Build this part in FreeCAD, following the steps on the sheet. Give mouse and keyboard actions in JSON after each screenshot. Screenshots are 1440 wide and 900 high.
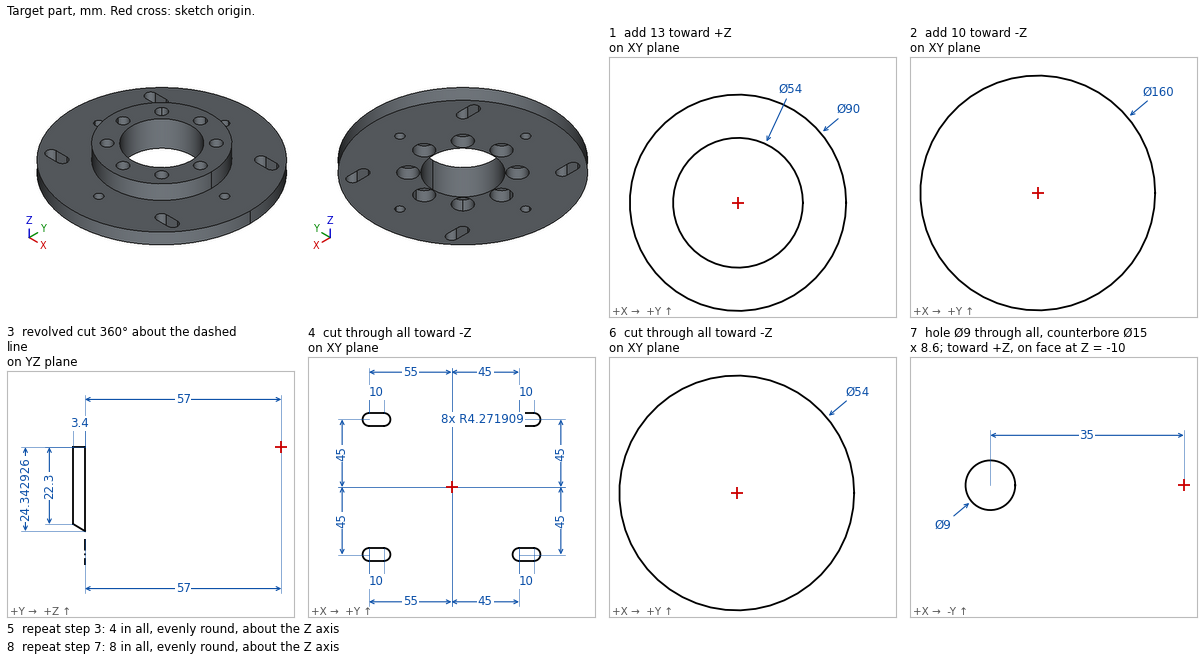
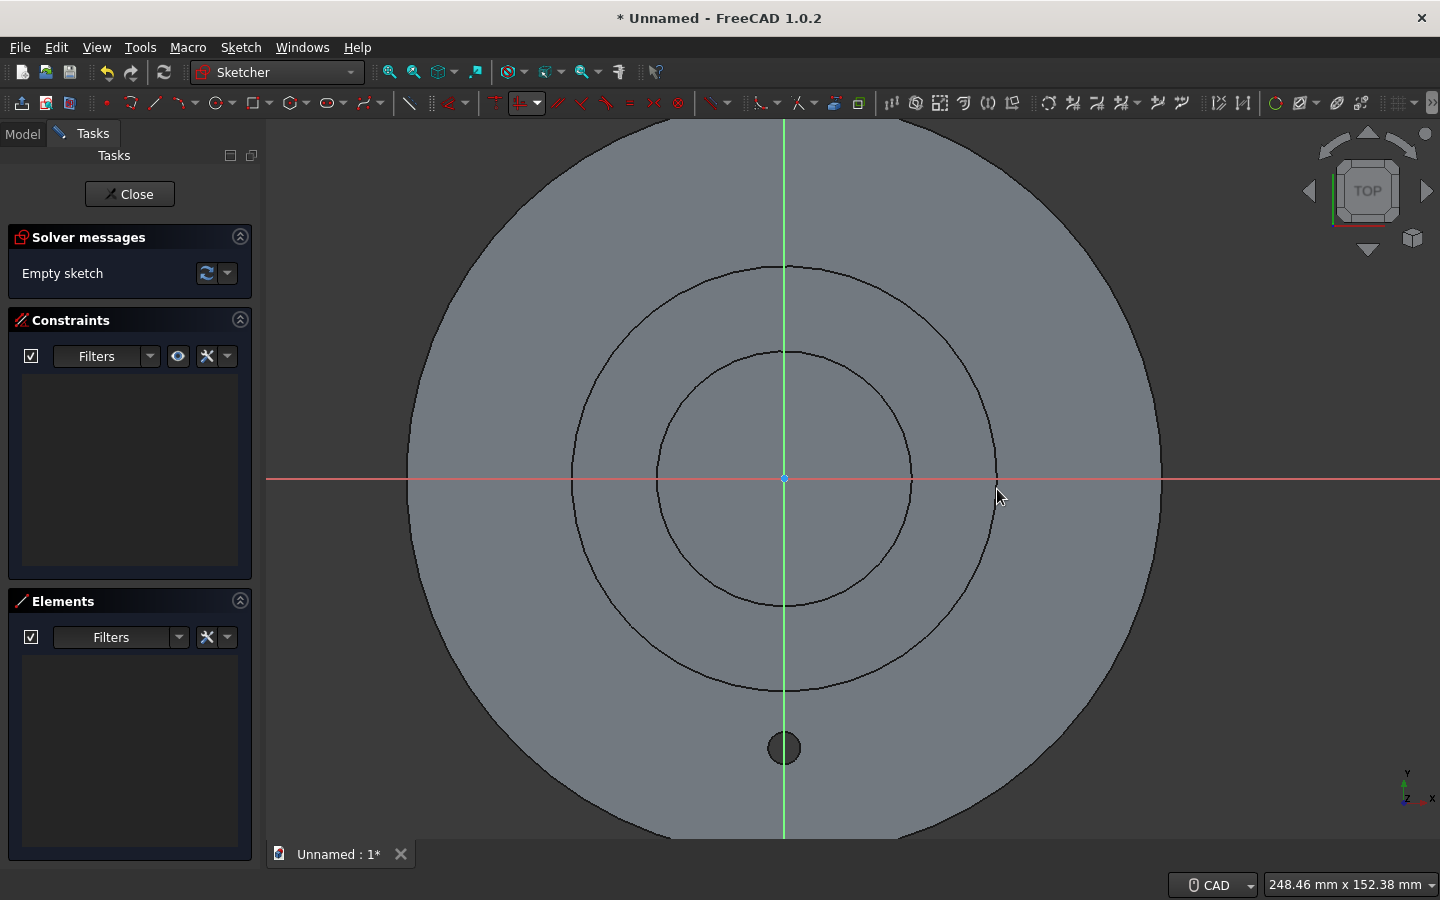
{"action": "left_click", "coordinate": [997, 266]}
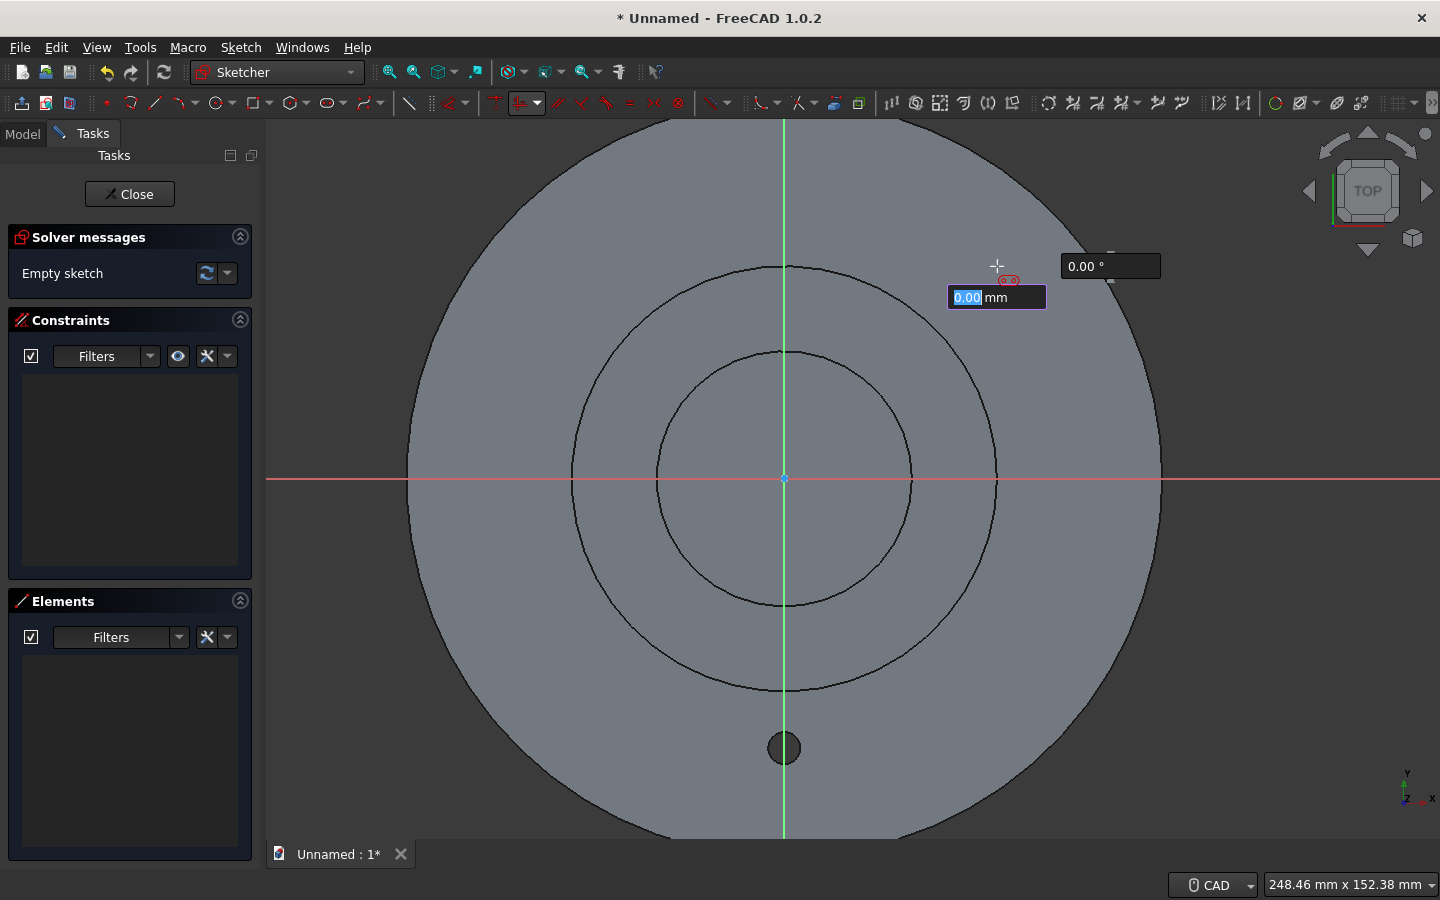
{"action": "left_click", "coordinate": [1044, 266]}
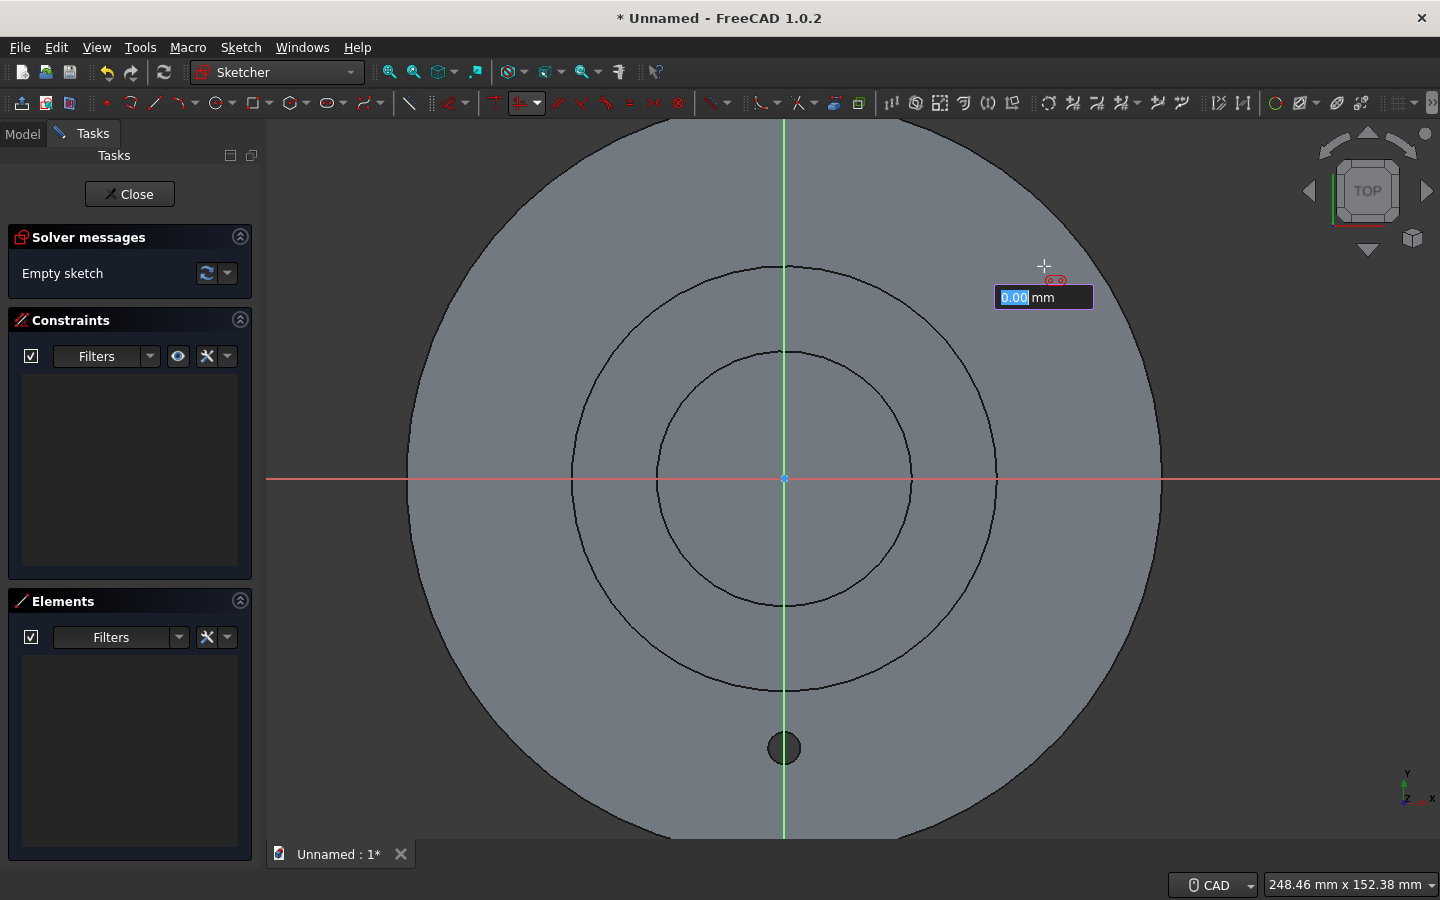
{"action": "left_click", "coordinate": [1021, 246]}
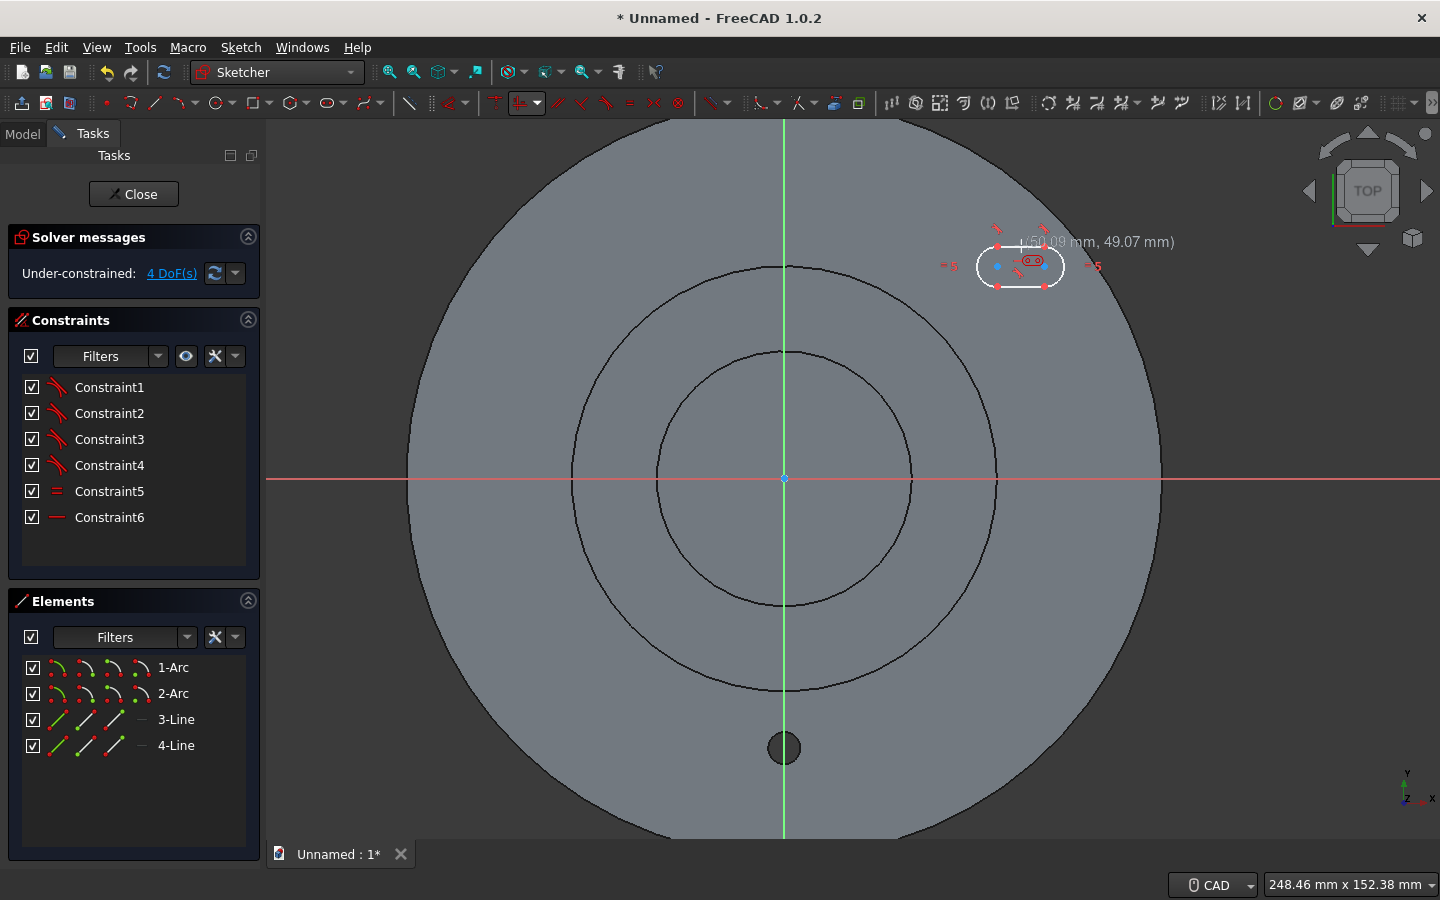
{"action": "left_click", "coordinate": [997, 691]}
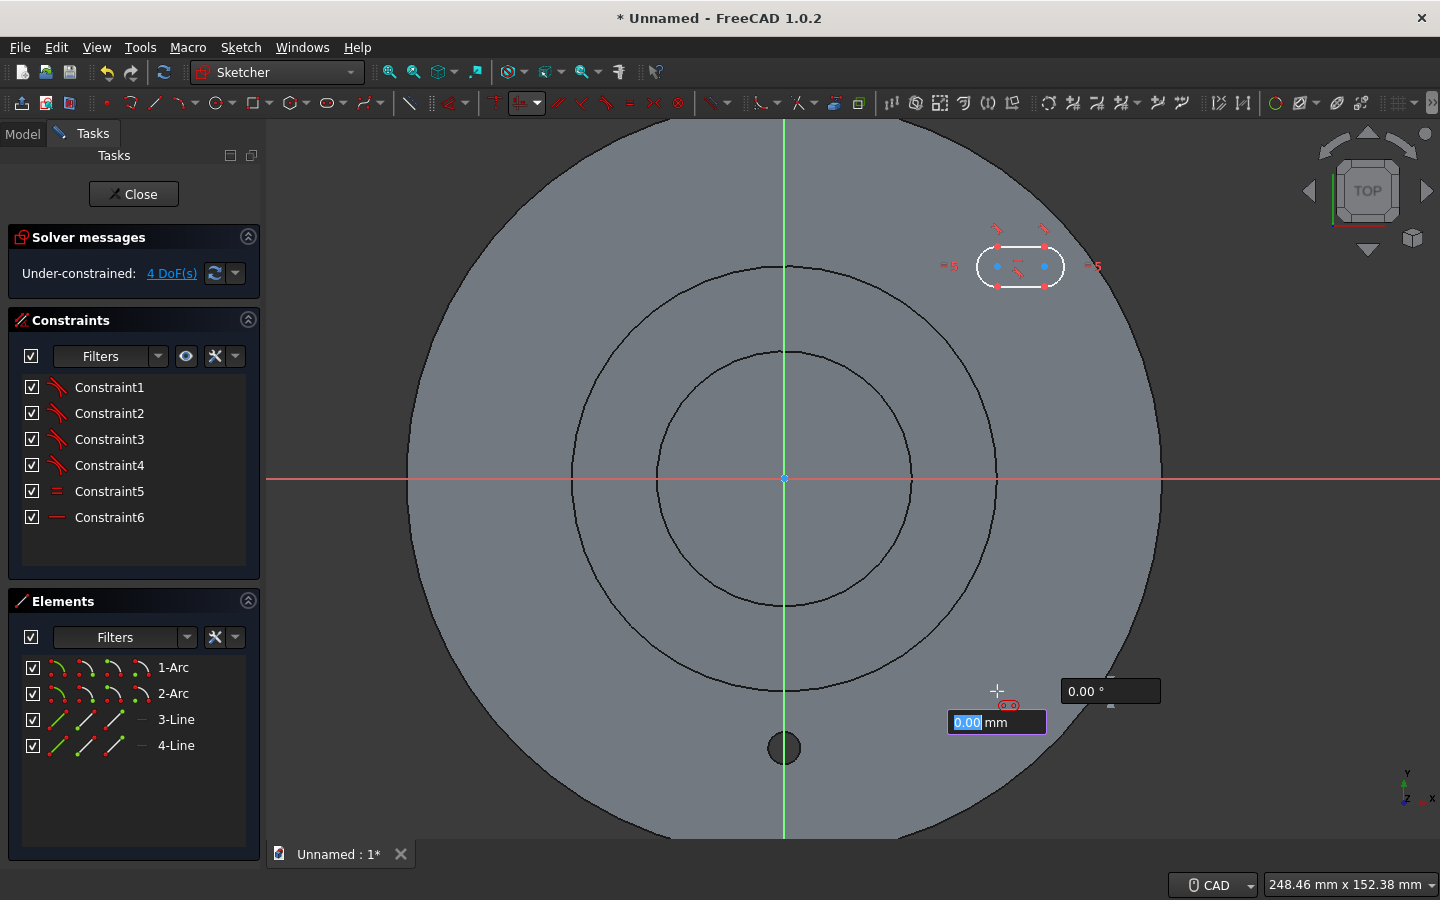
{"action": "left_click", "coordinate": [1044, 691]}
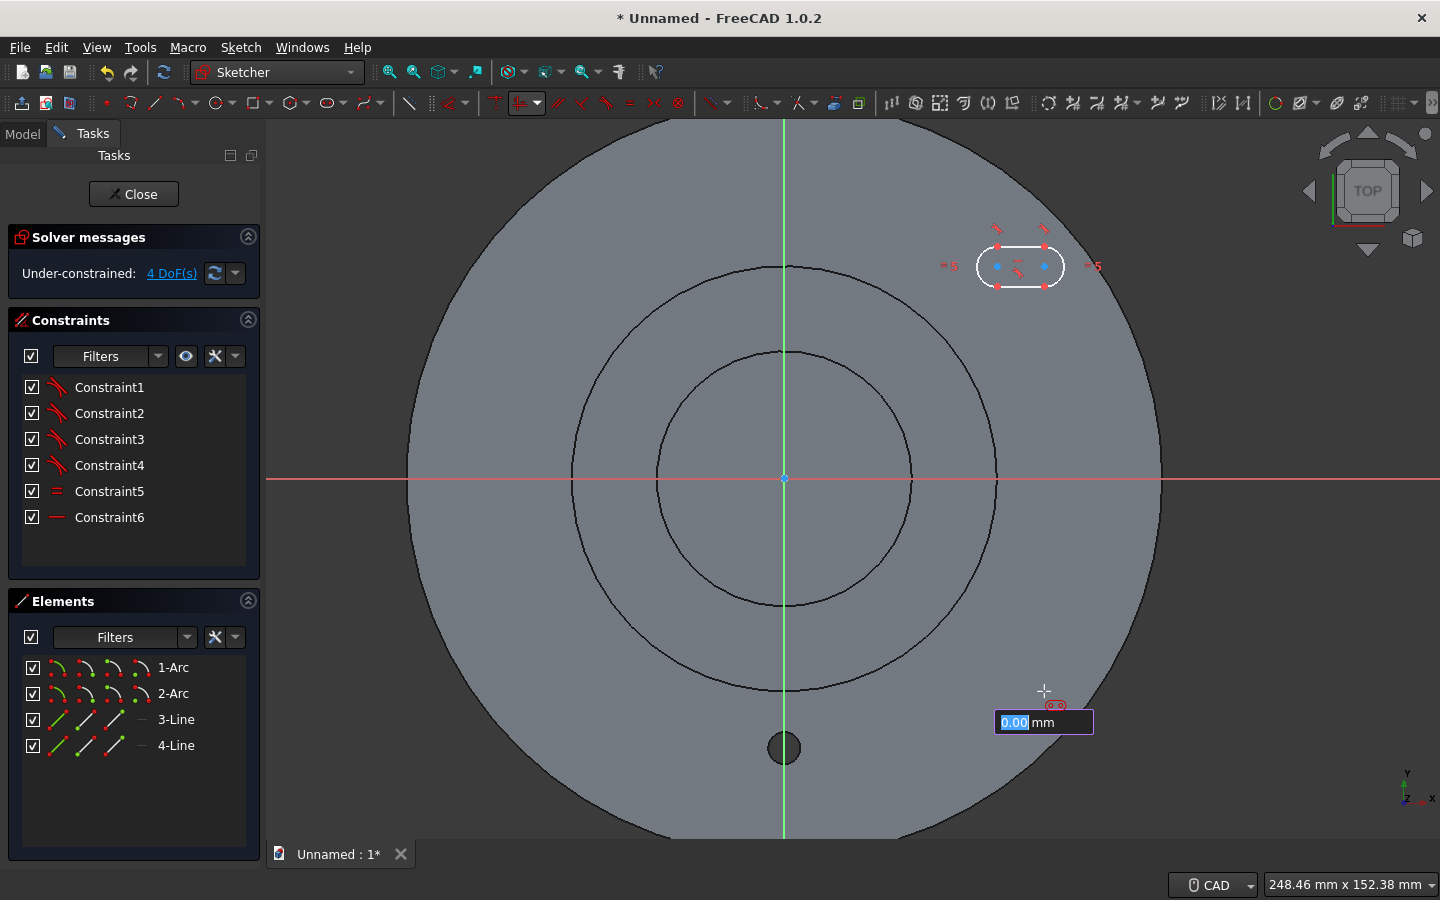
{"action": "left_click", "coordinate": [1021, 671]}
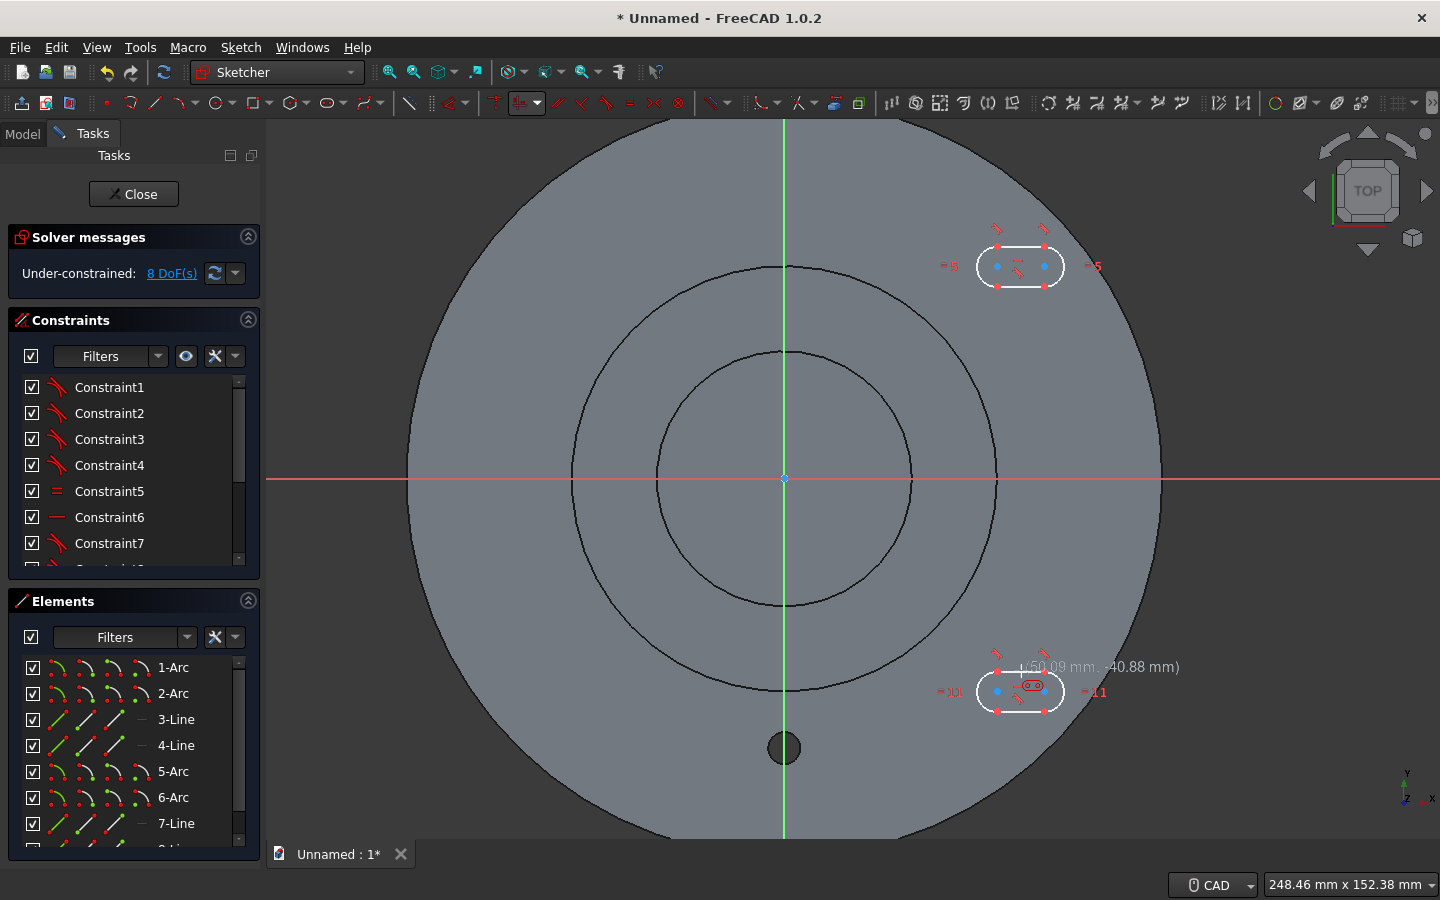
{"action": "left_click", "coordinate": [524, 691]}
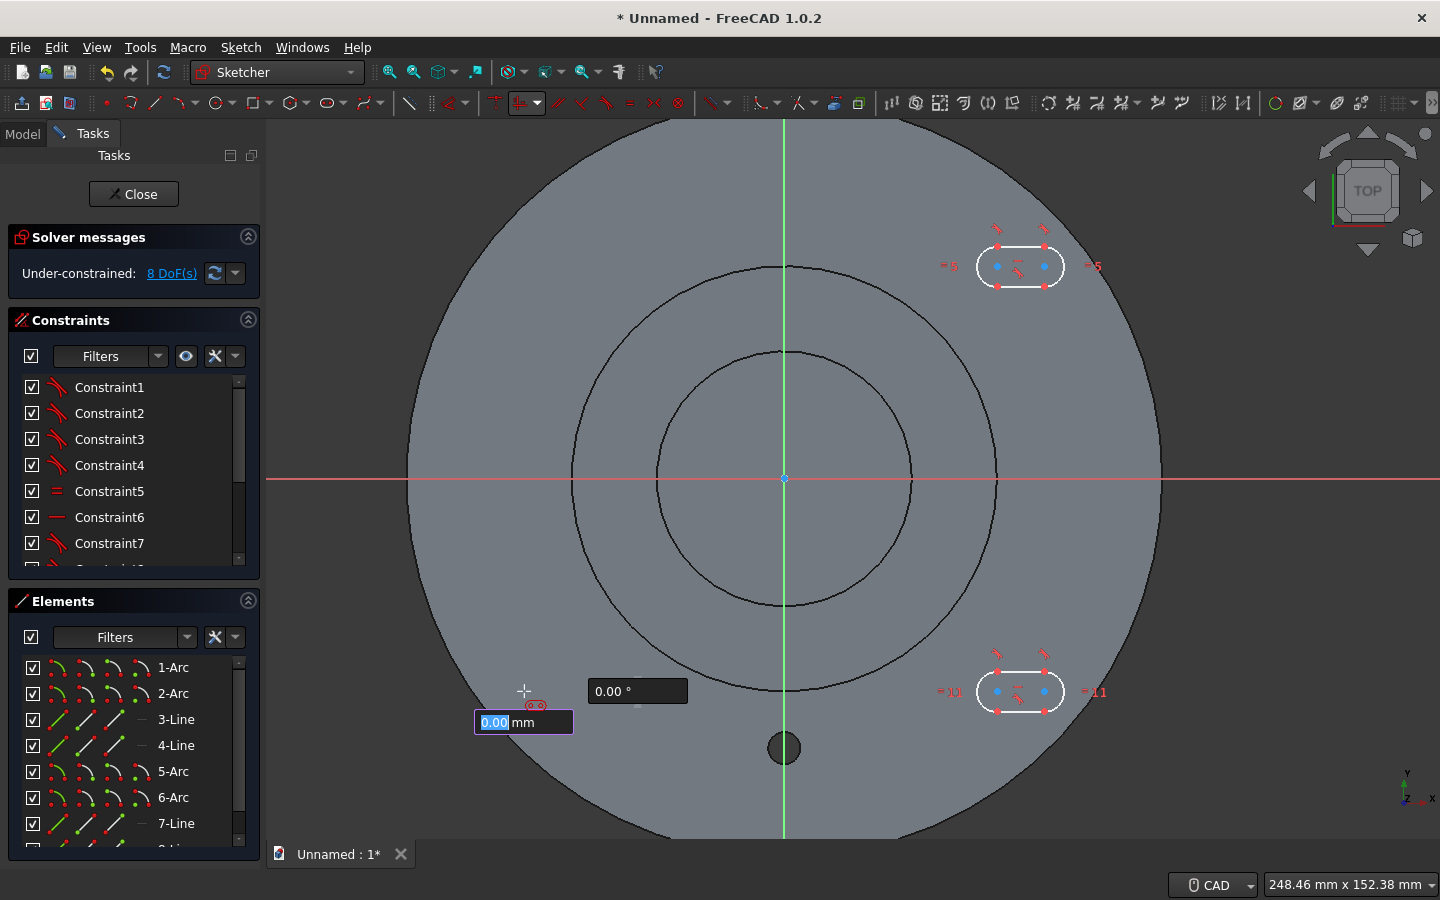
{"action": "left_click", "coordinate": [572, 691]}